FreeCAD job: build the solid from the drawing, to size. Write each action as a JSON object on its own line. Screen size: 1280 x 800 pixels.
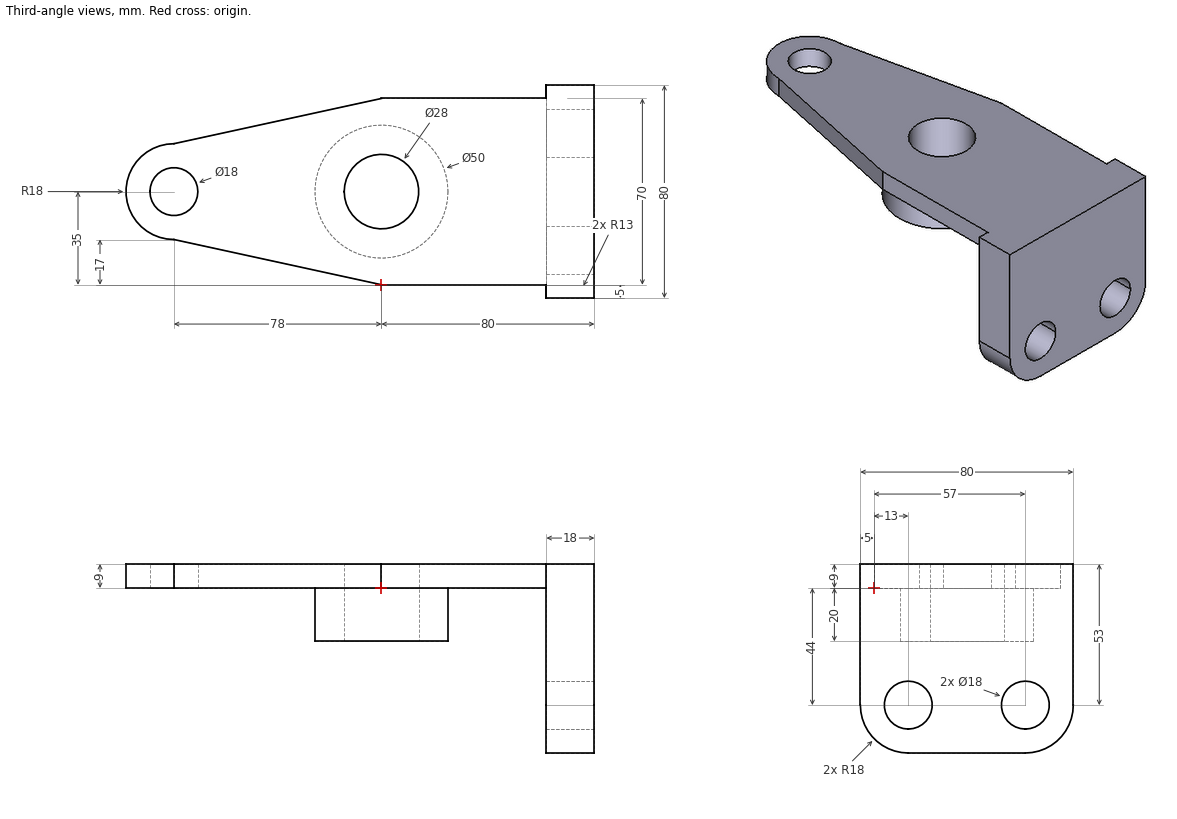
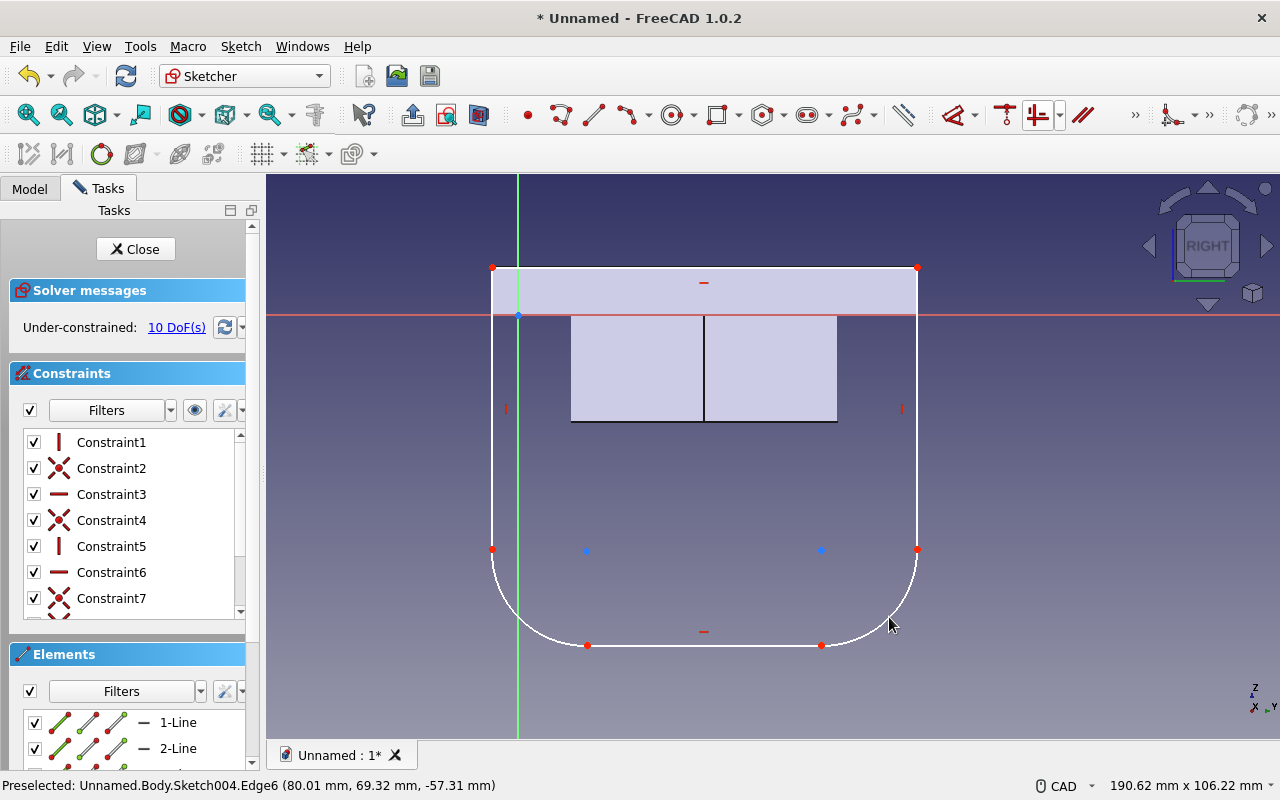
{"action": "left_click", "coordinate": [917, 465]}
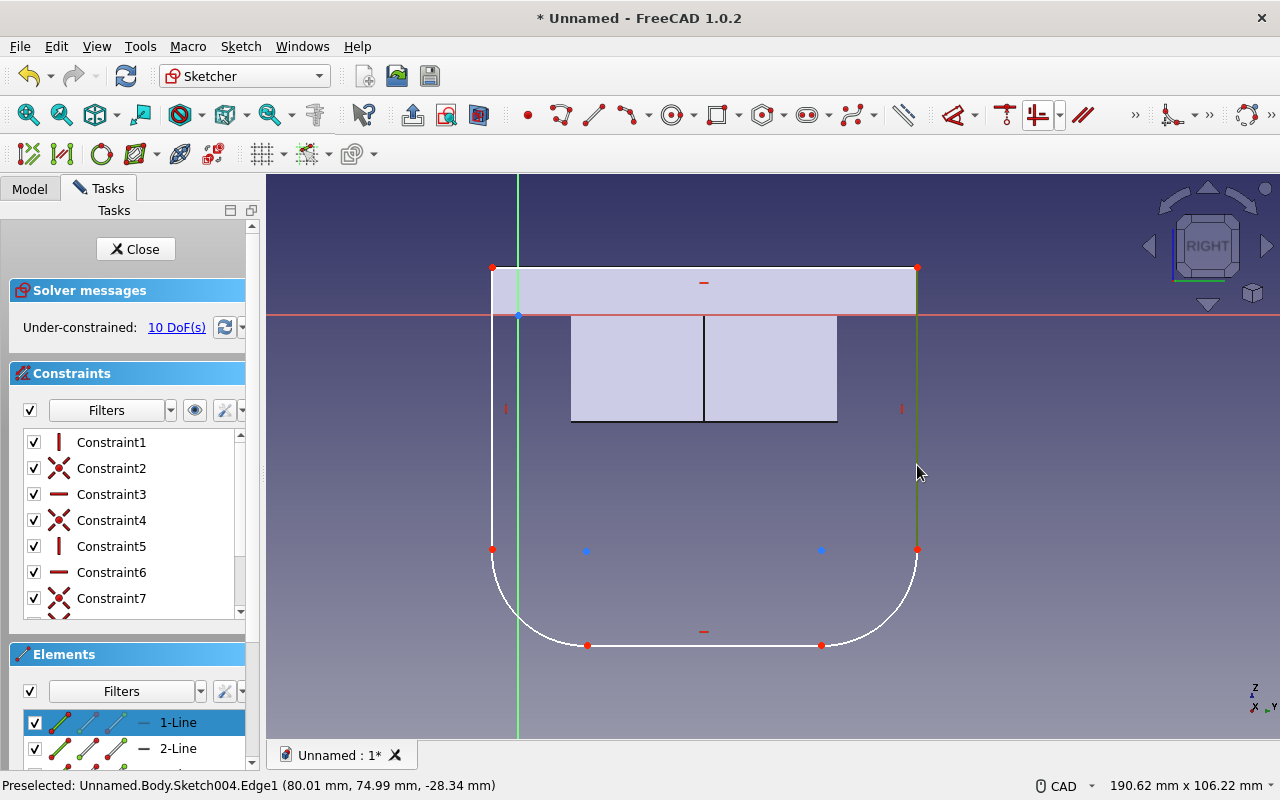
{"action": "left_click", "coordinate": [865, 636]}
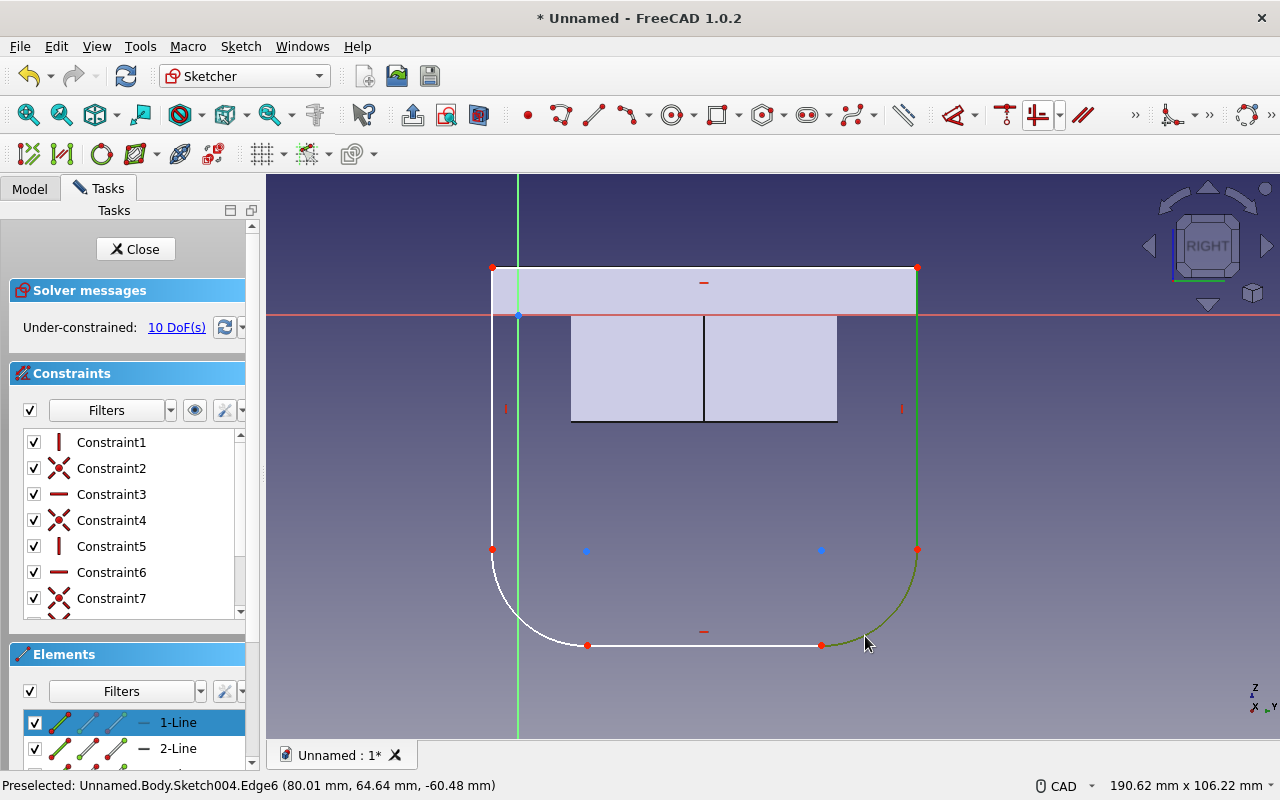
{"action": "key", "text": "t"}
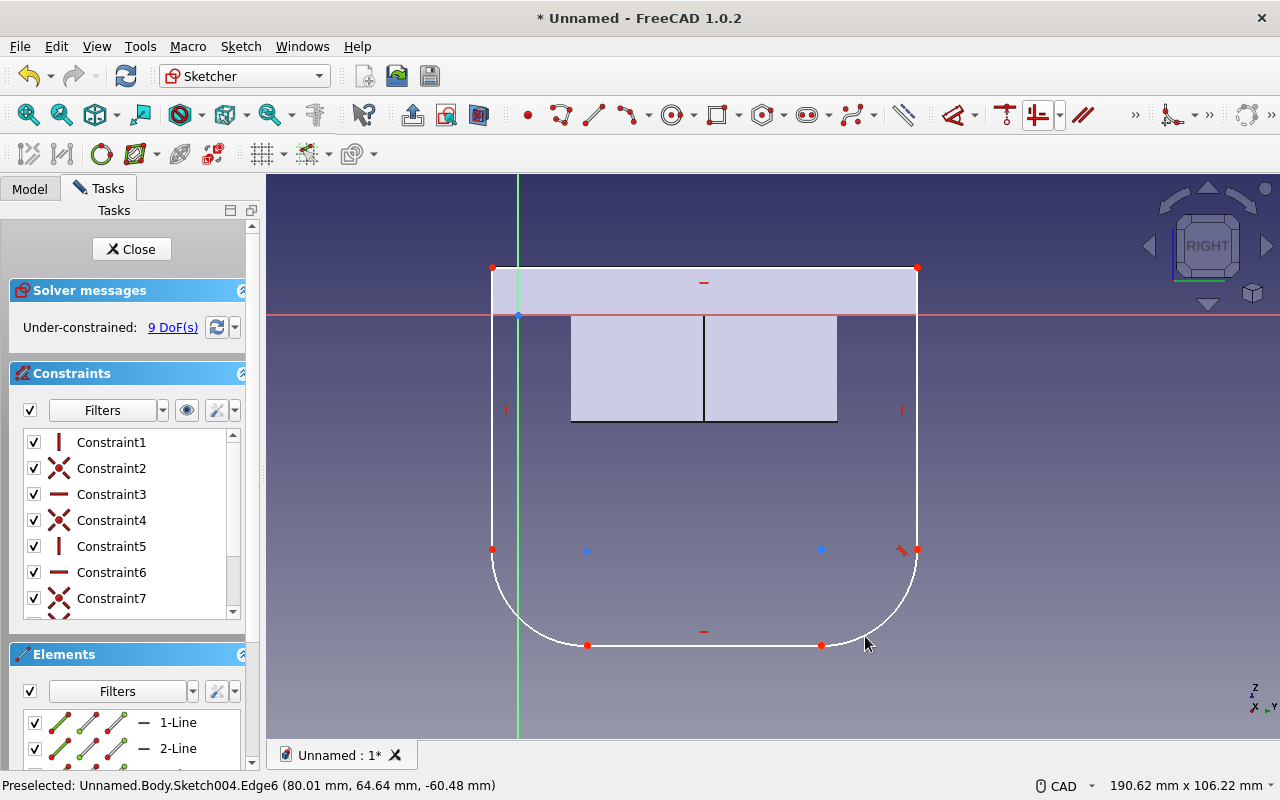
{"action": "left_click", "coordinate": [492, 353]}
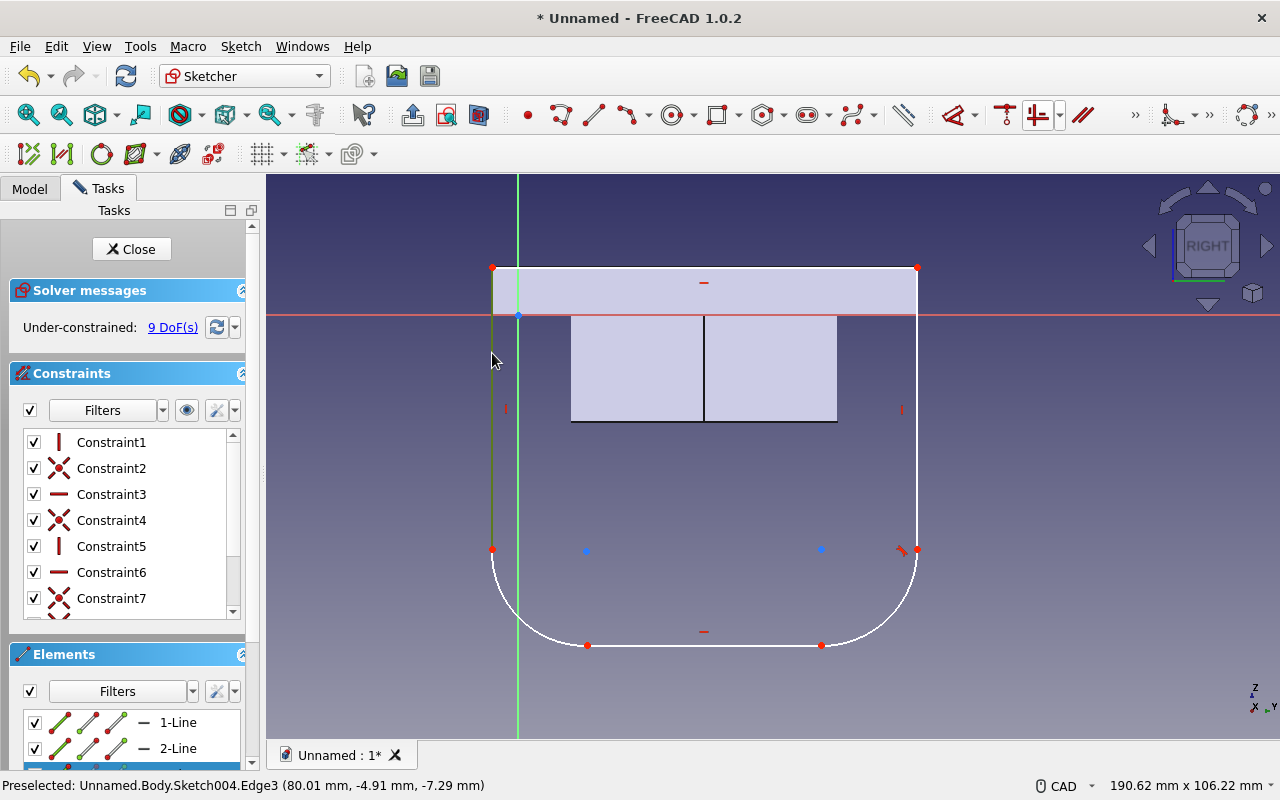
{"action": "left_click", "coordinate": [502, 594]}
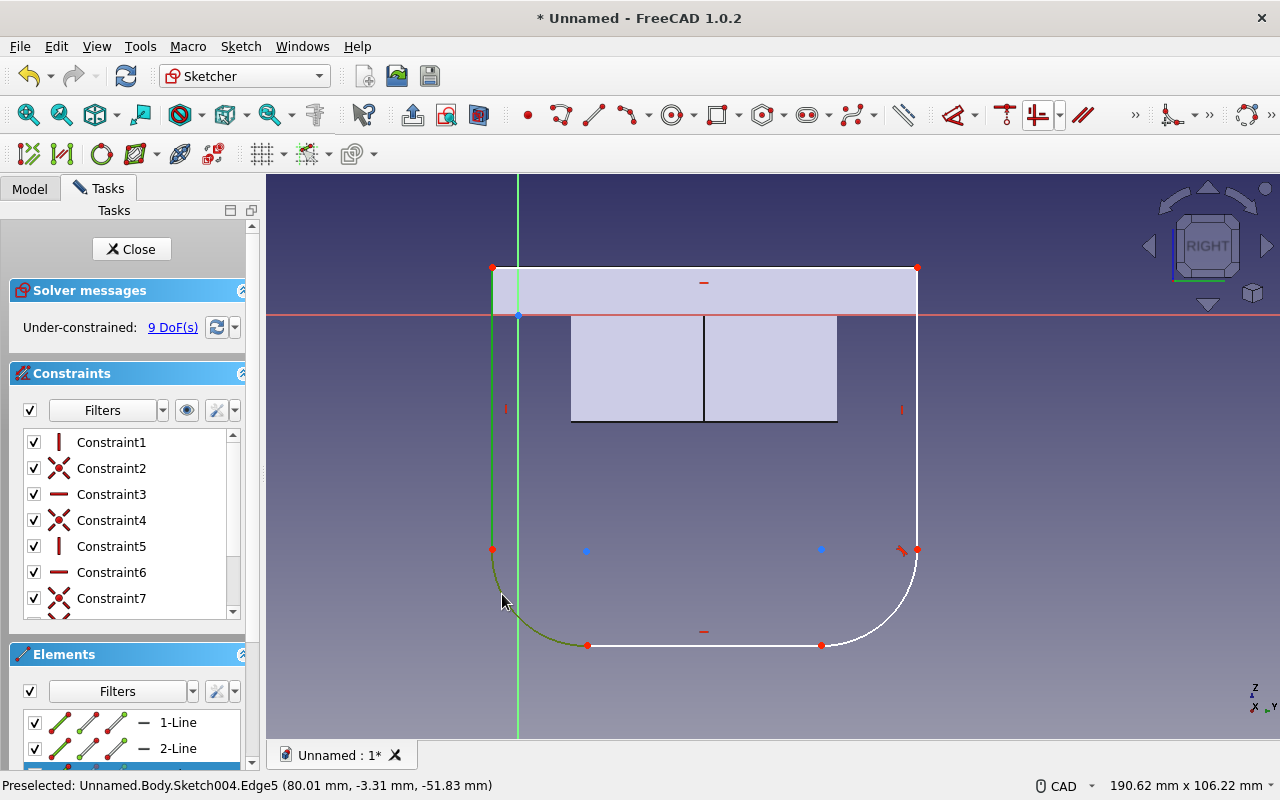
{"action": "key", "text": "t"}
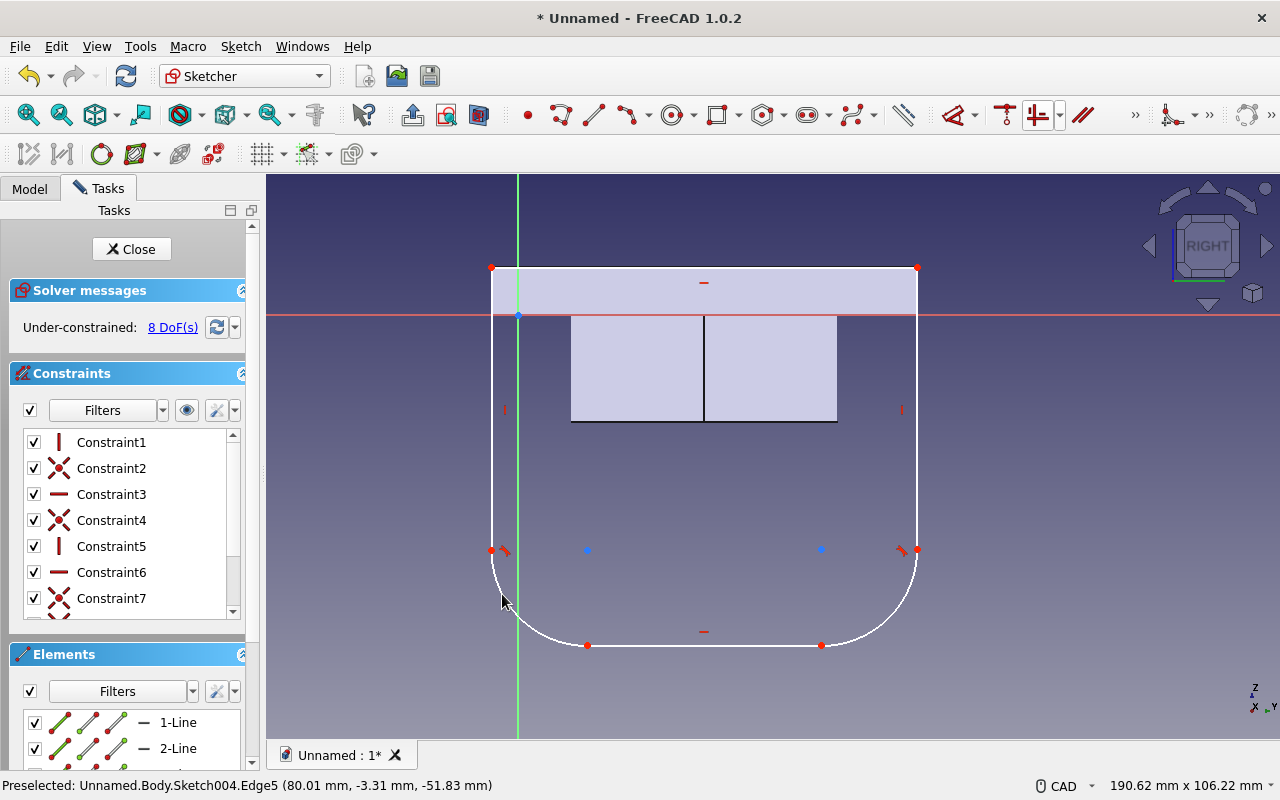
{"action": "left_click", "coordinate": [657, 646]}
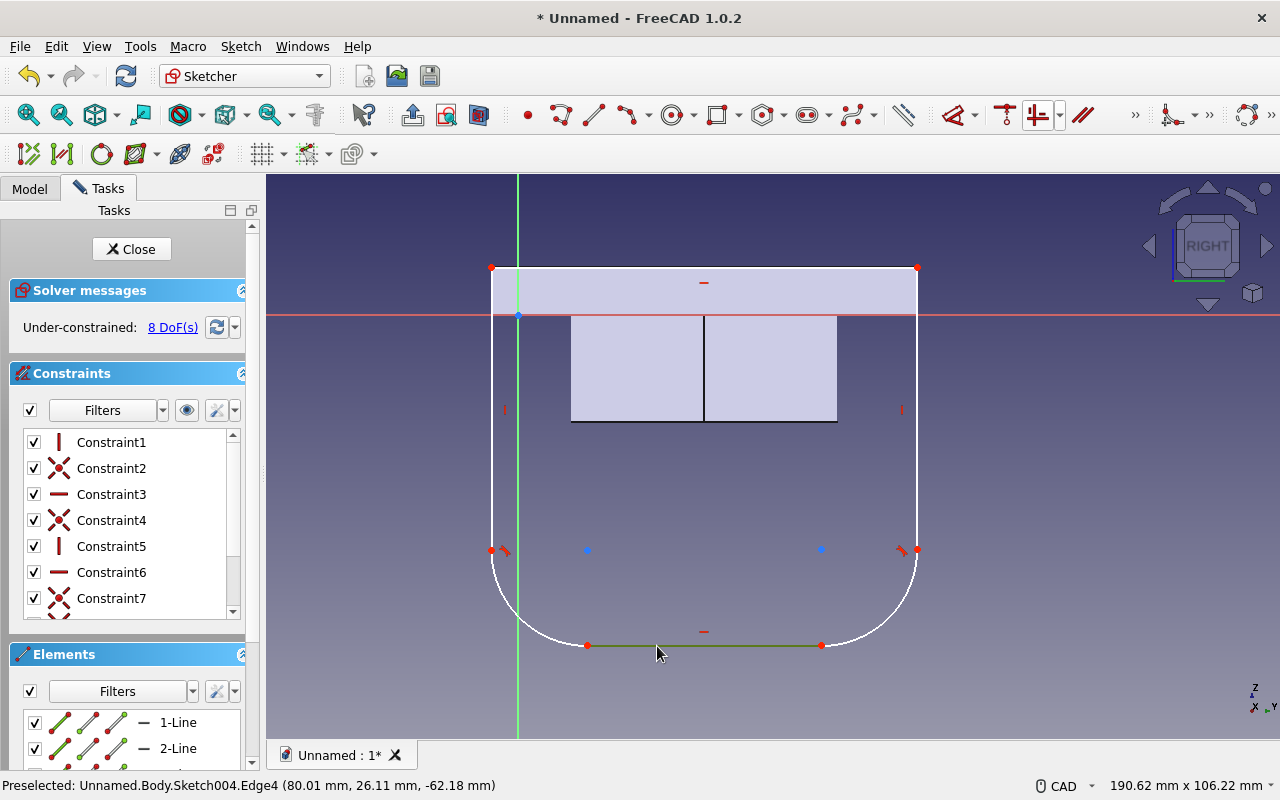
{"action": "left_click", "coordinate": [502, 593]}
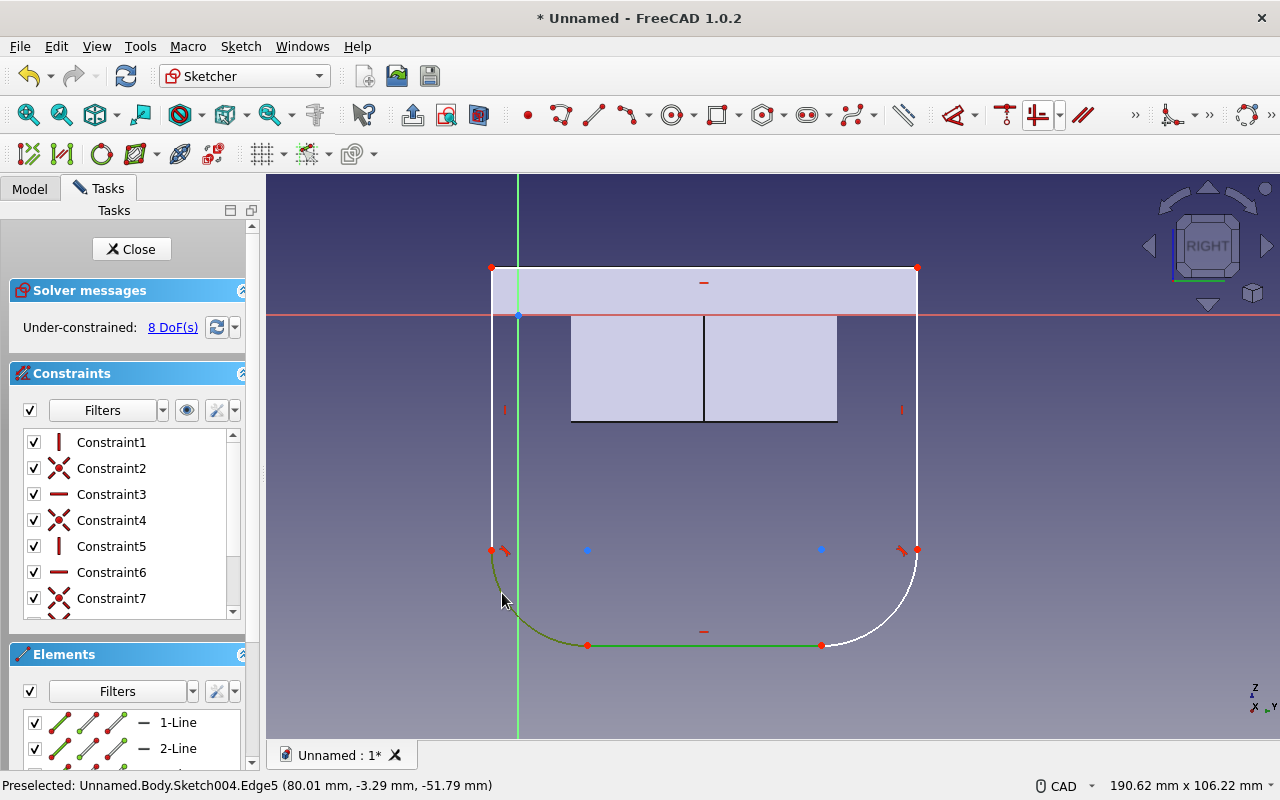
{"action": "key", "text": "t"}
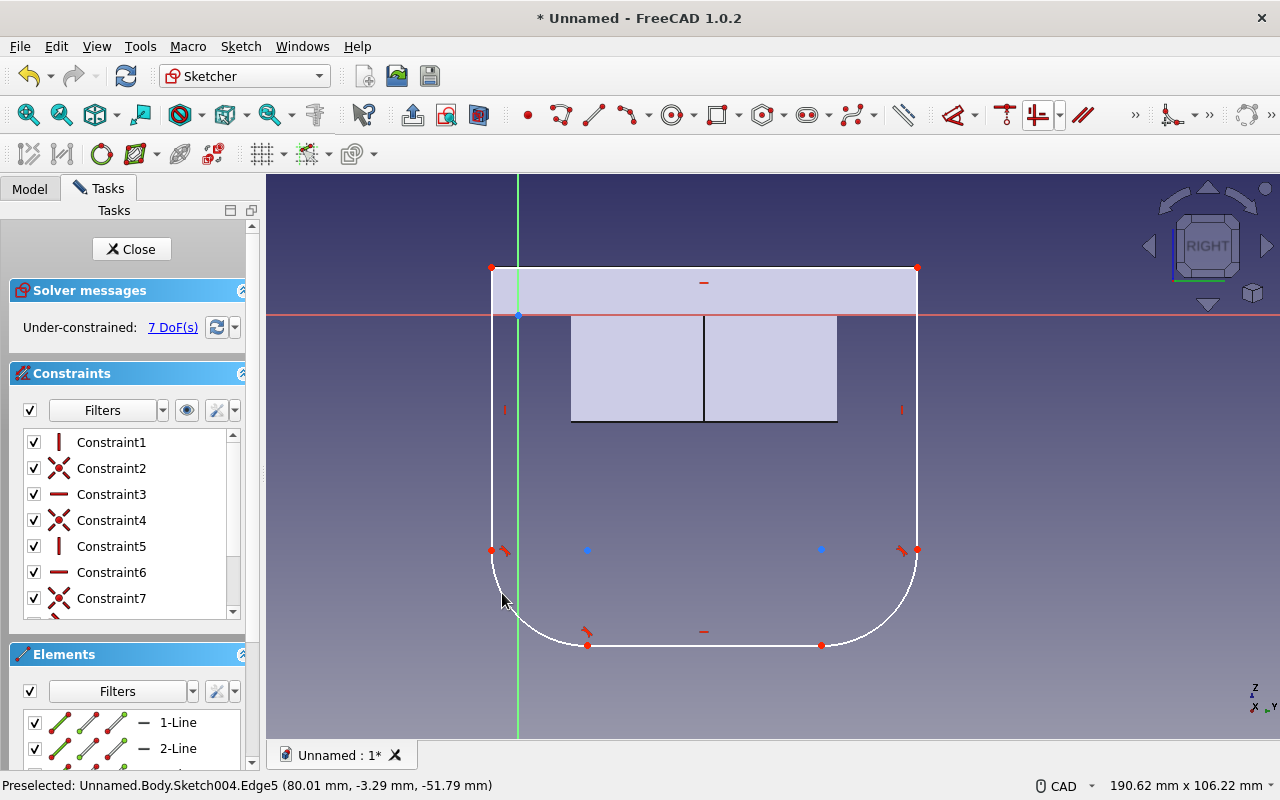
{"action": "left_click", "coordinate": [658, 646]}